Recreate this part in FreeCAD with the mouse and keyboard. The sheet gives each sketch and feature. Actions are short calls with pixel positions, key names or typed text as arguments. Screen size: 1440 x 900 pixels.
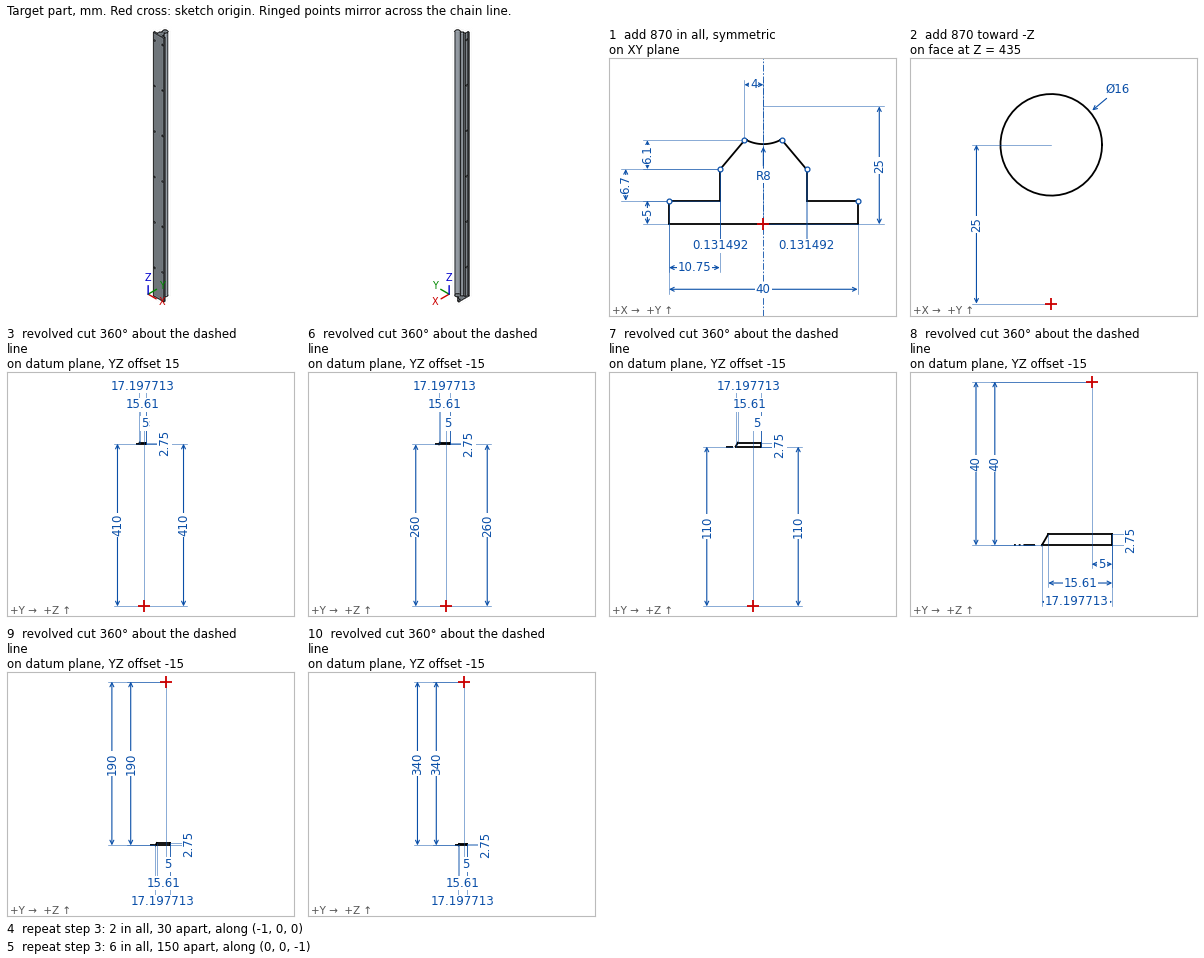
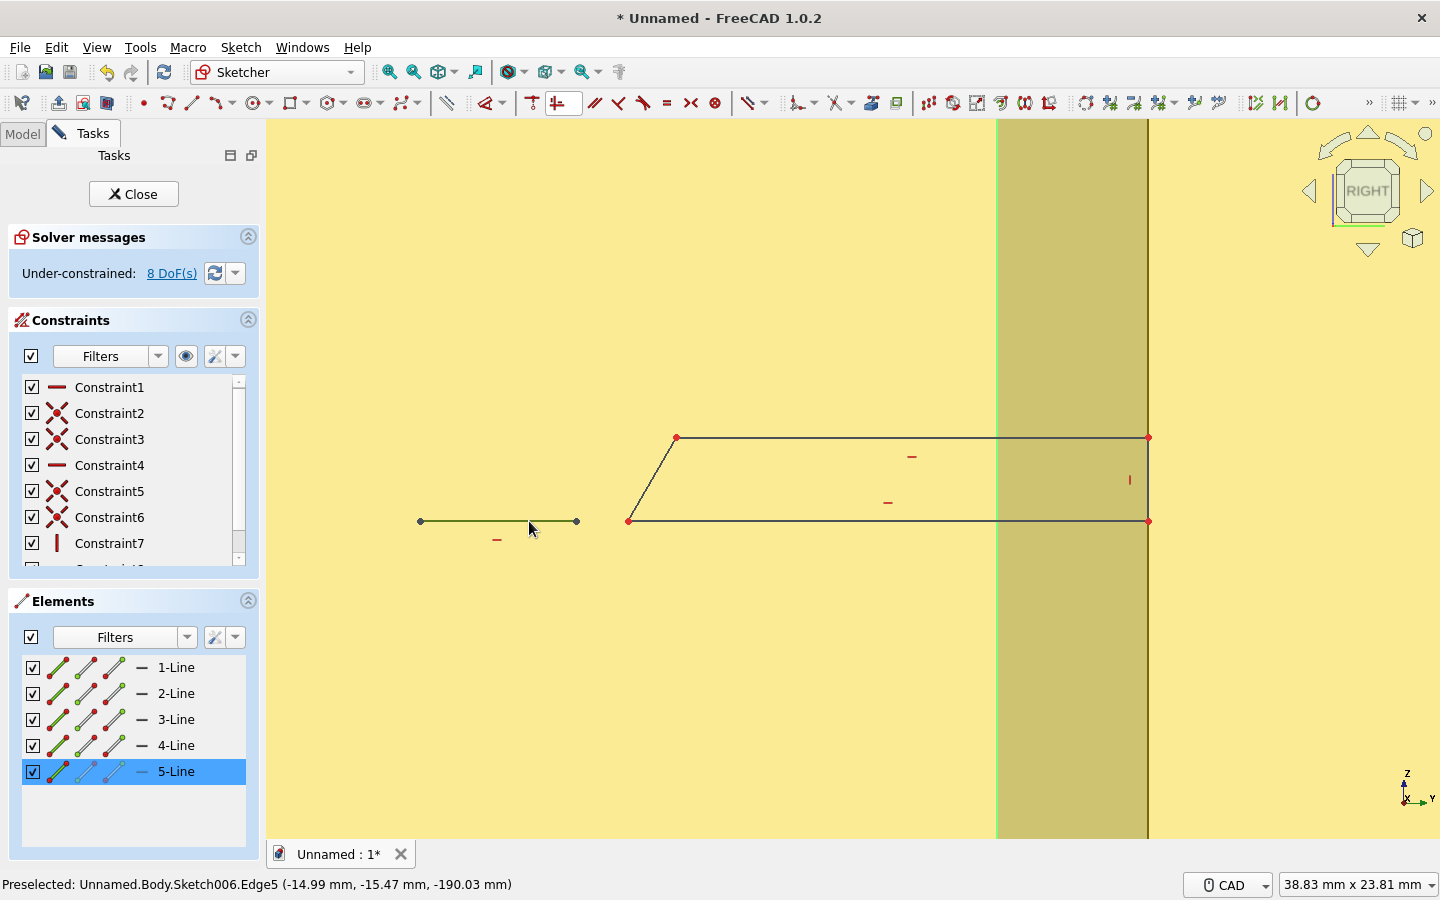
click(448, 104)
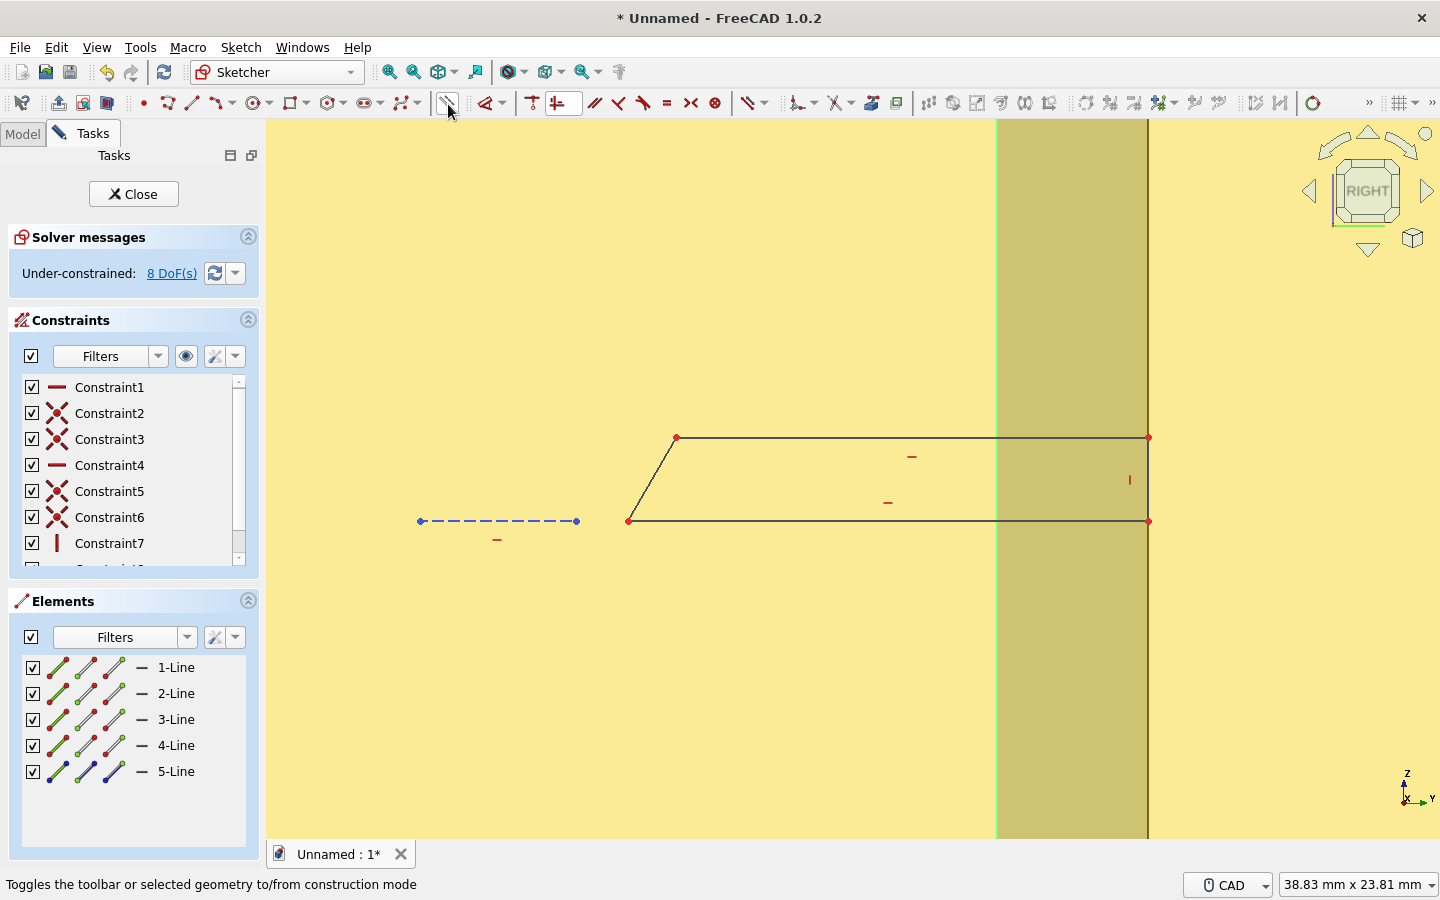
click(486, 104)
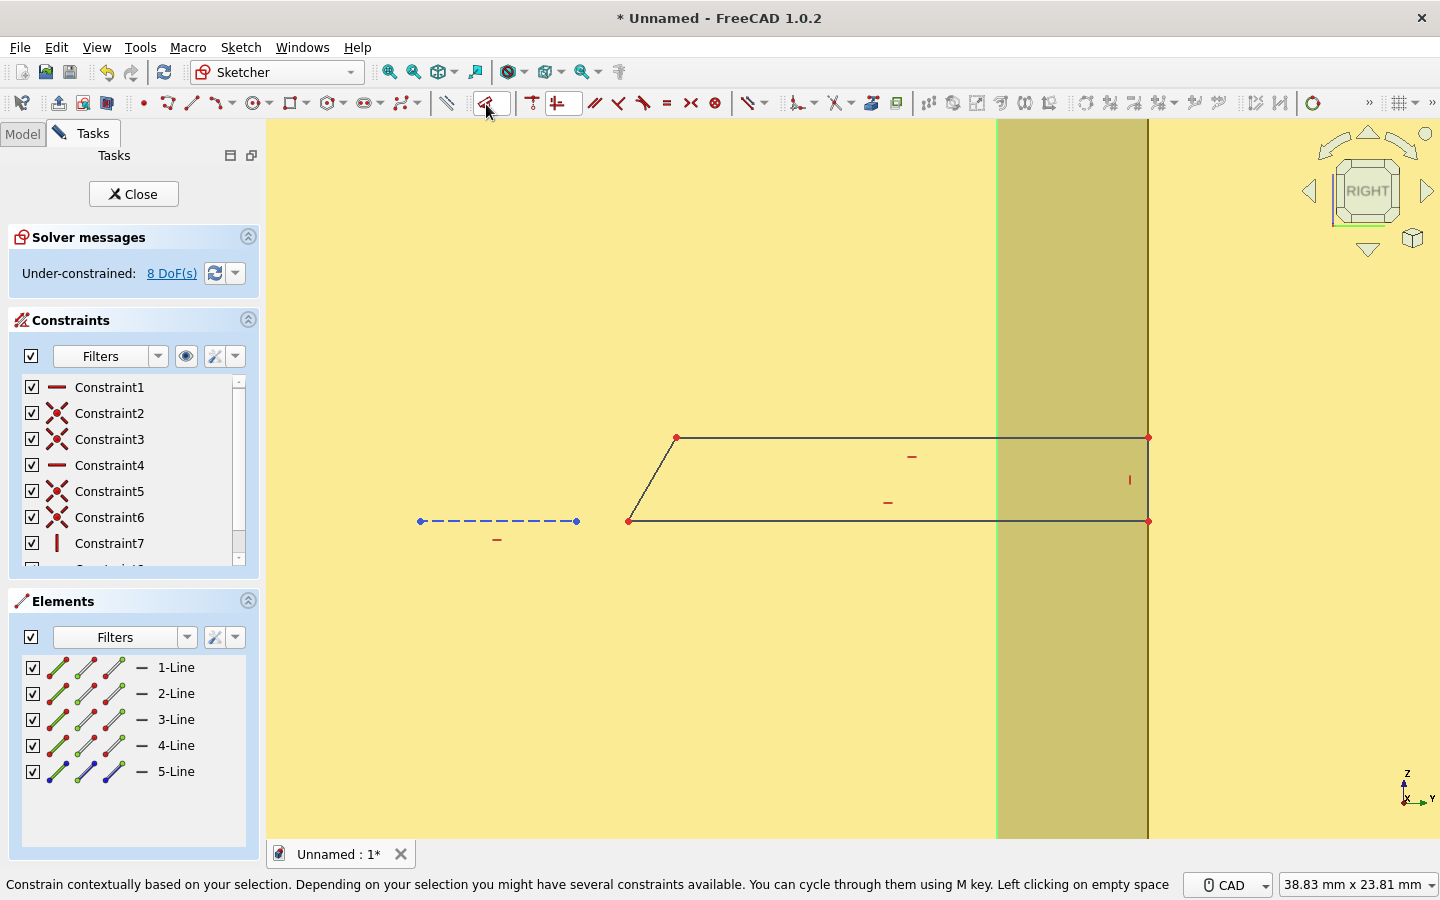
click(1148, 438)
click(1072, 472)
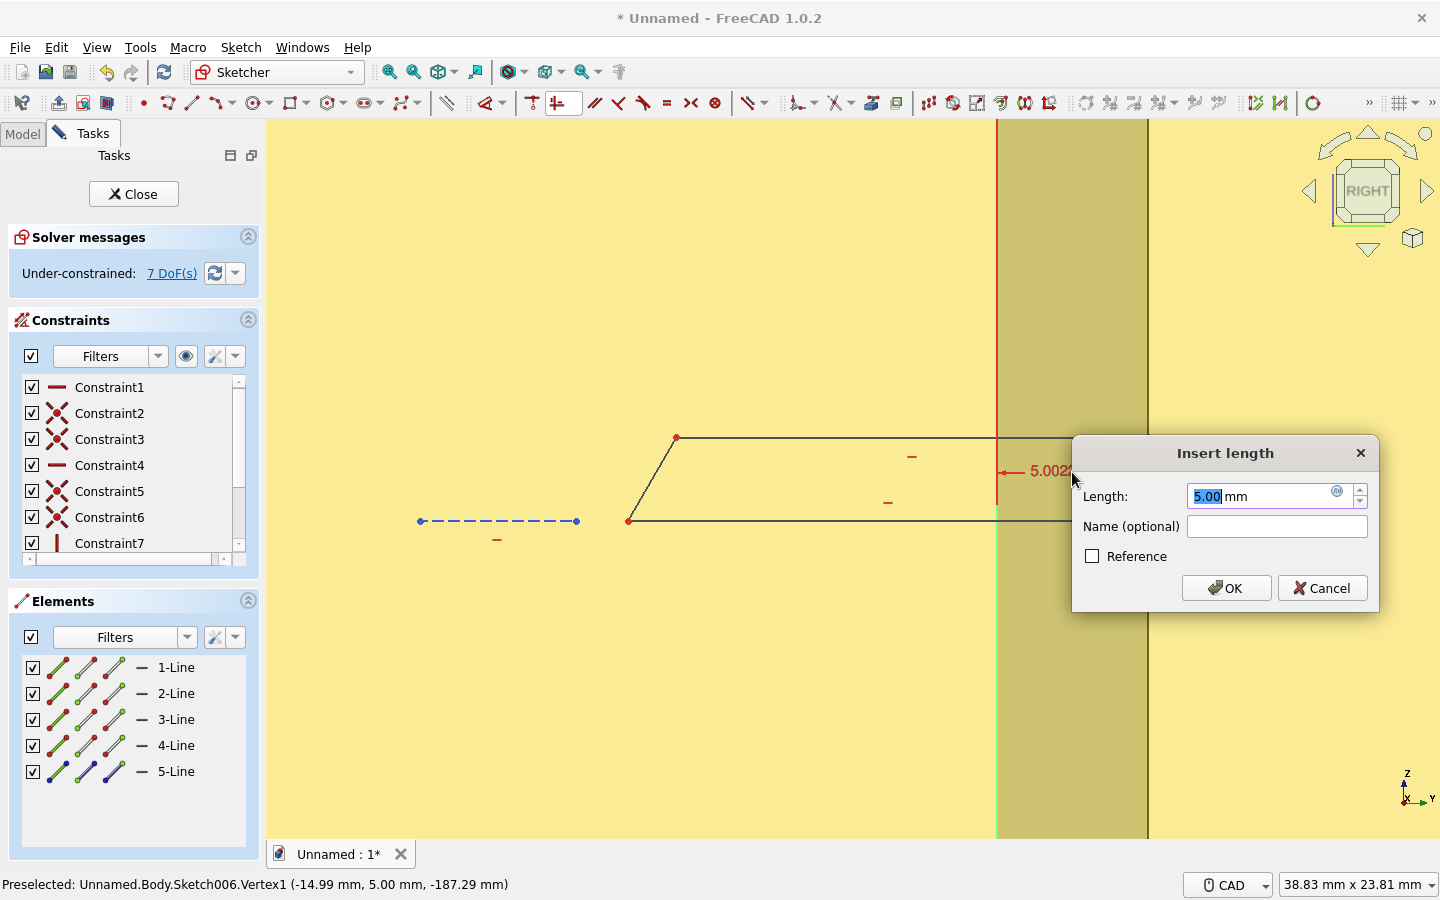
text(5)
key(Return)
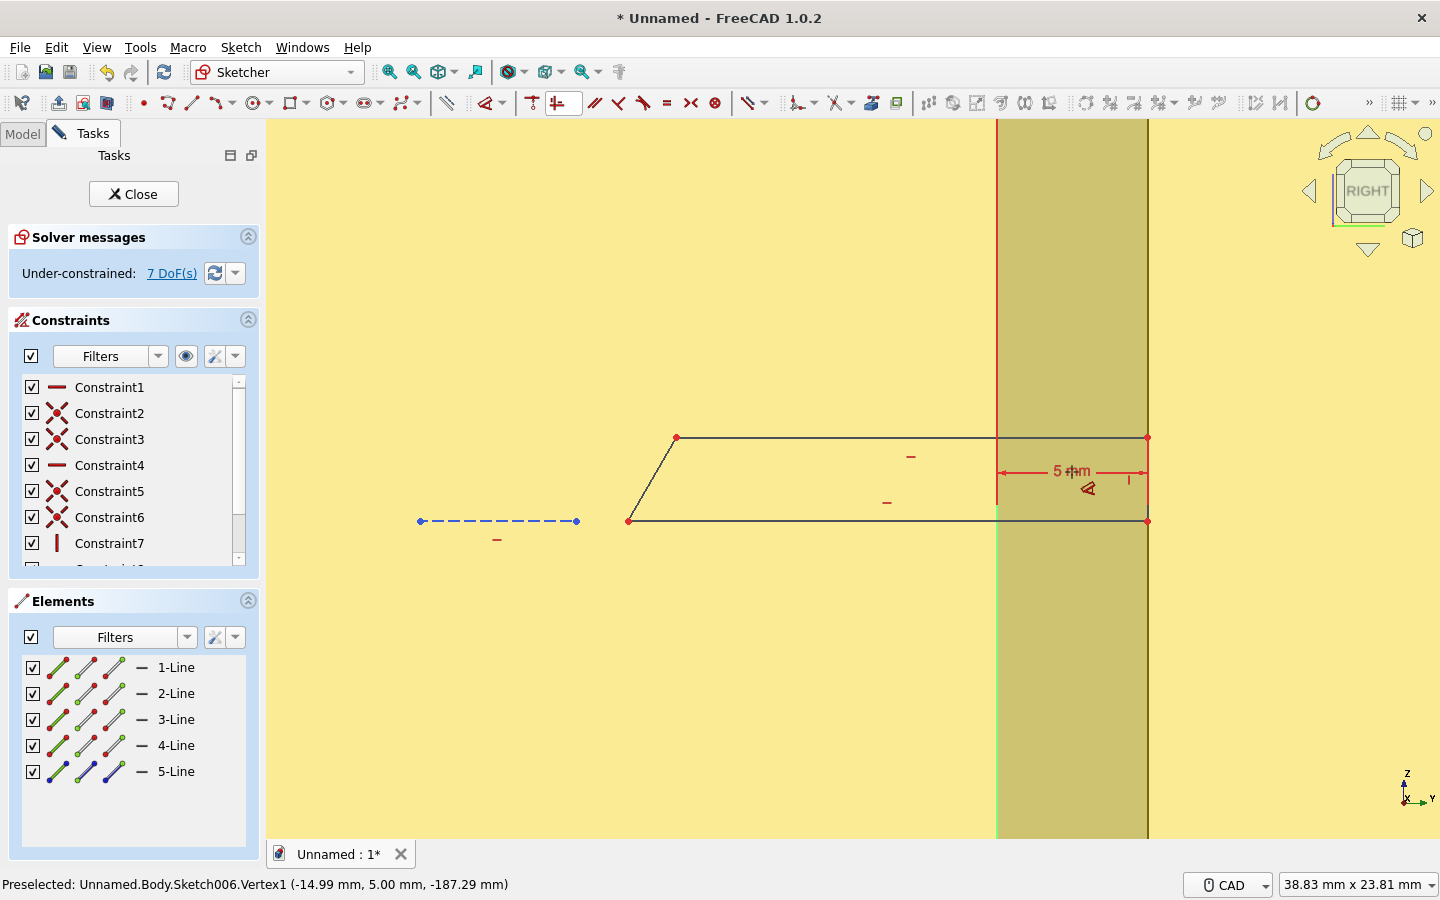
click(1148, 496)
click(1182, 480)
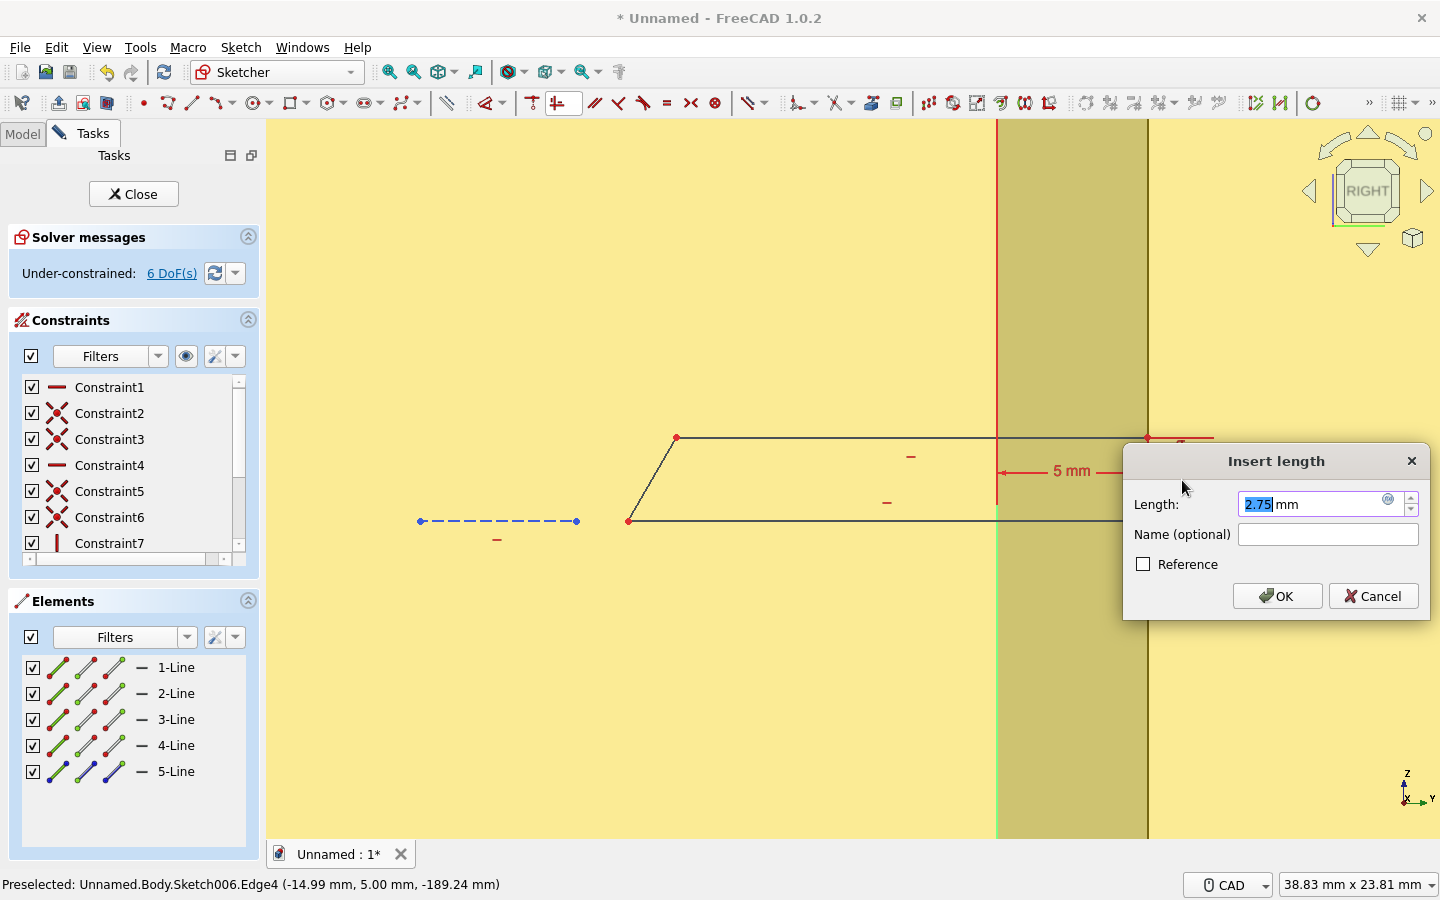
text(2.75)
key(Return)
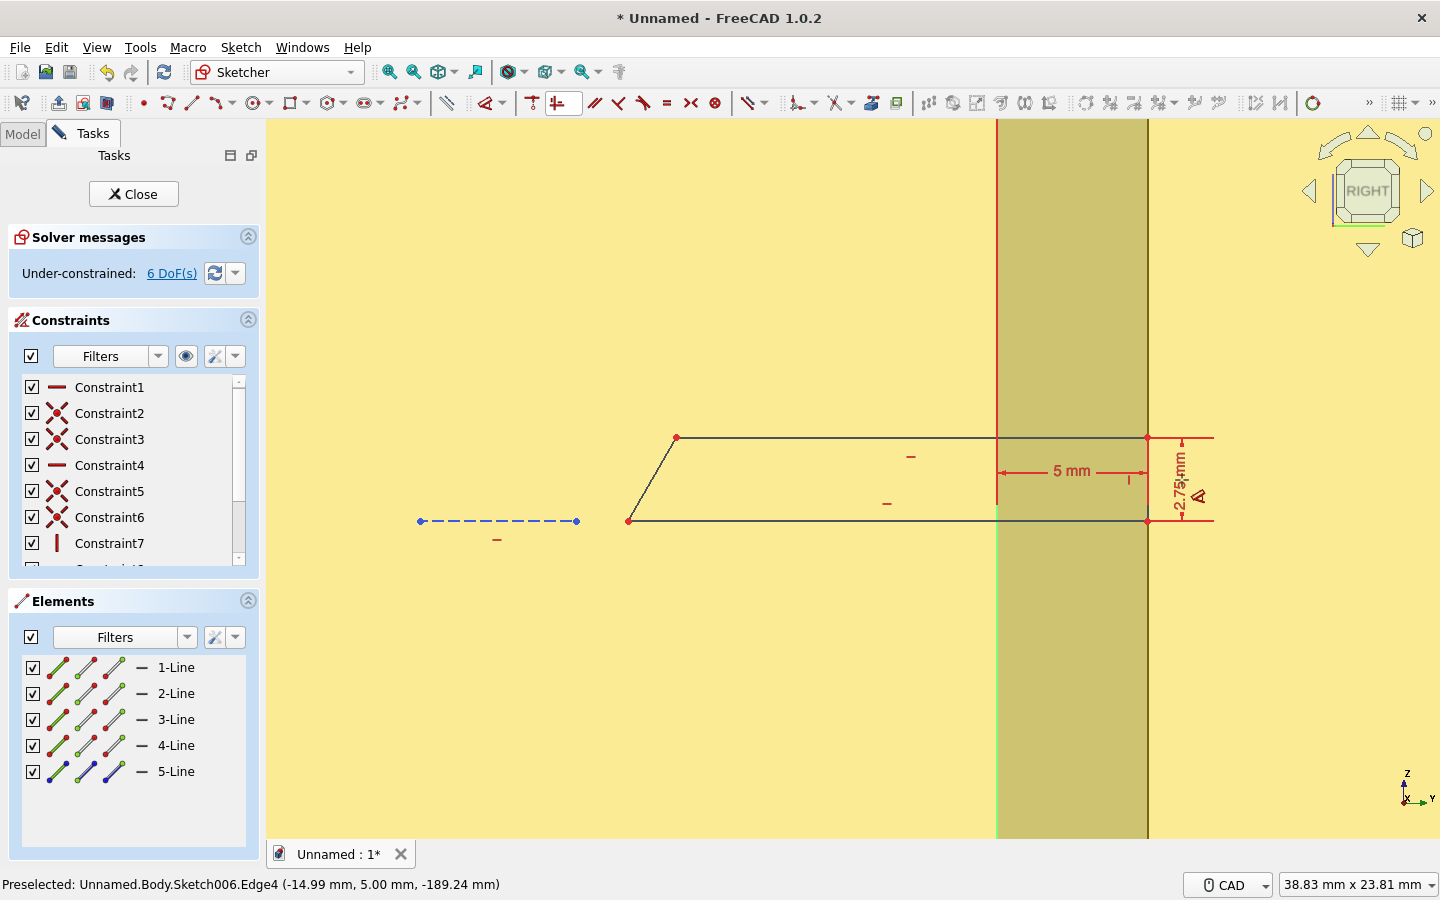
click(628, 521)
click(1031, 334)